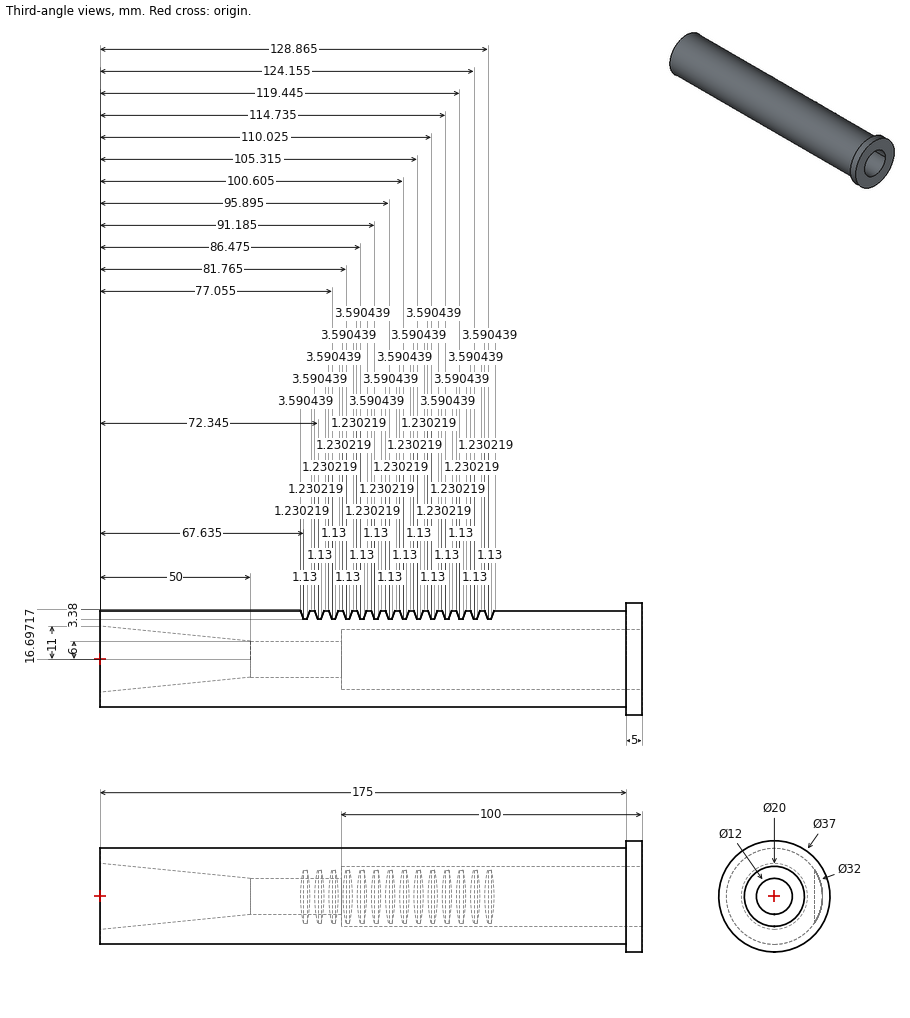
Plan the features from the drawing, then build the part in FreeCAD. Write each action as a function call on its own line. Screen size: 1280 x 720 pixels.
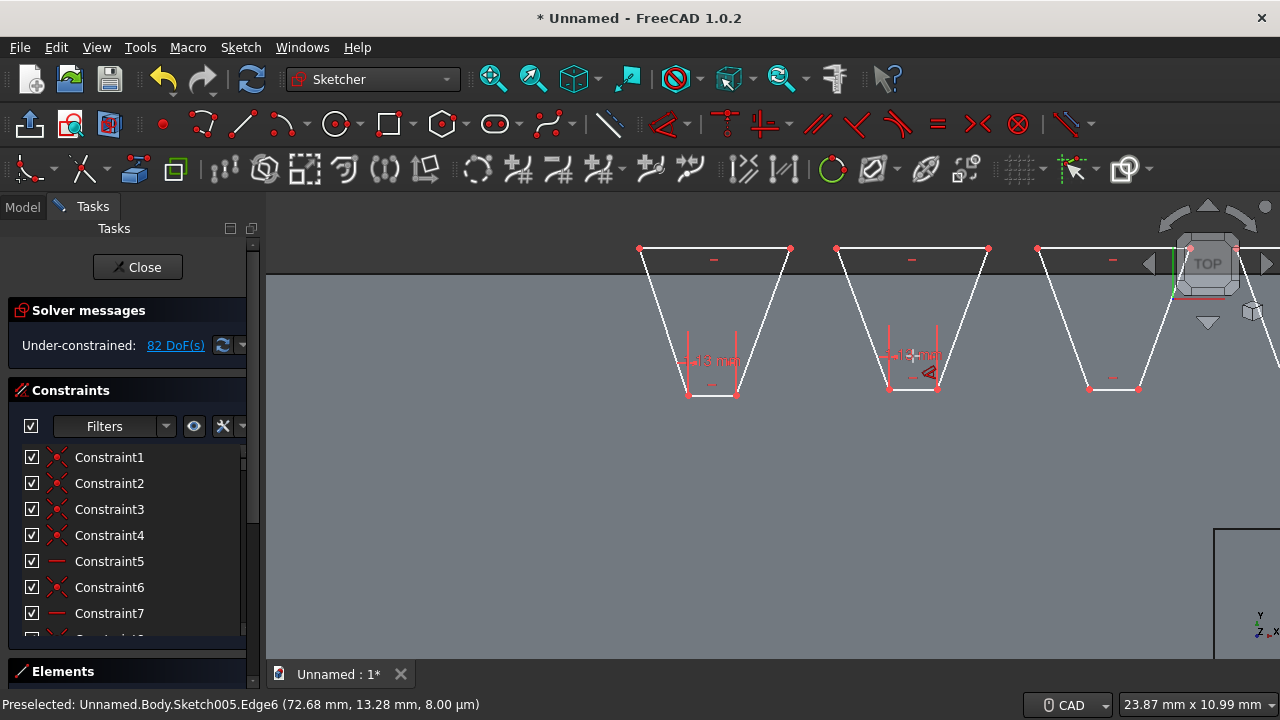
click(1104, 390)
click(1102, 356)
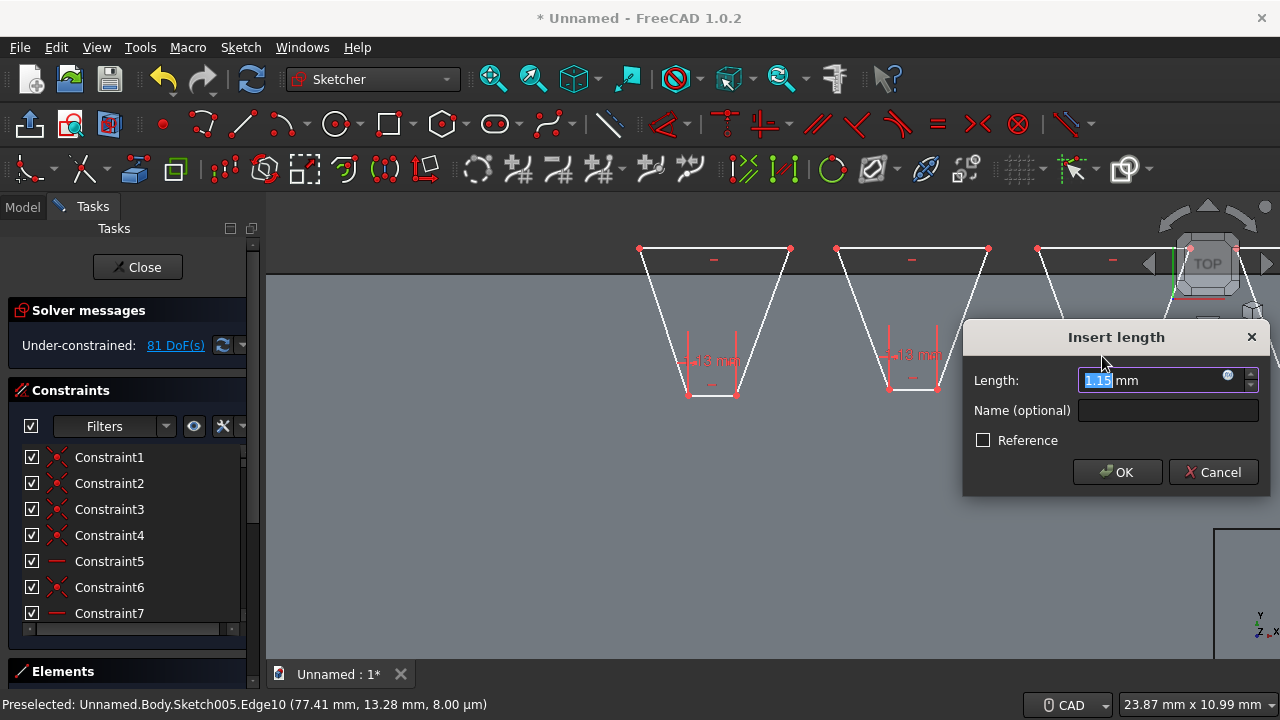
text(1.13)
key(Return)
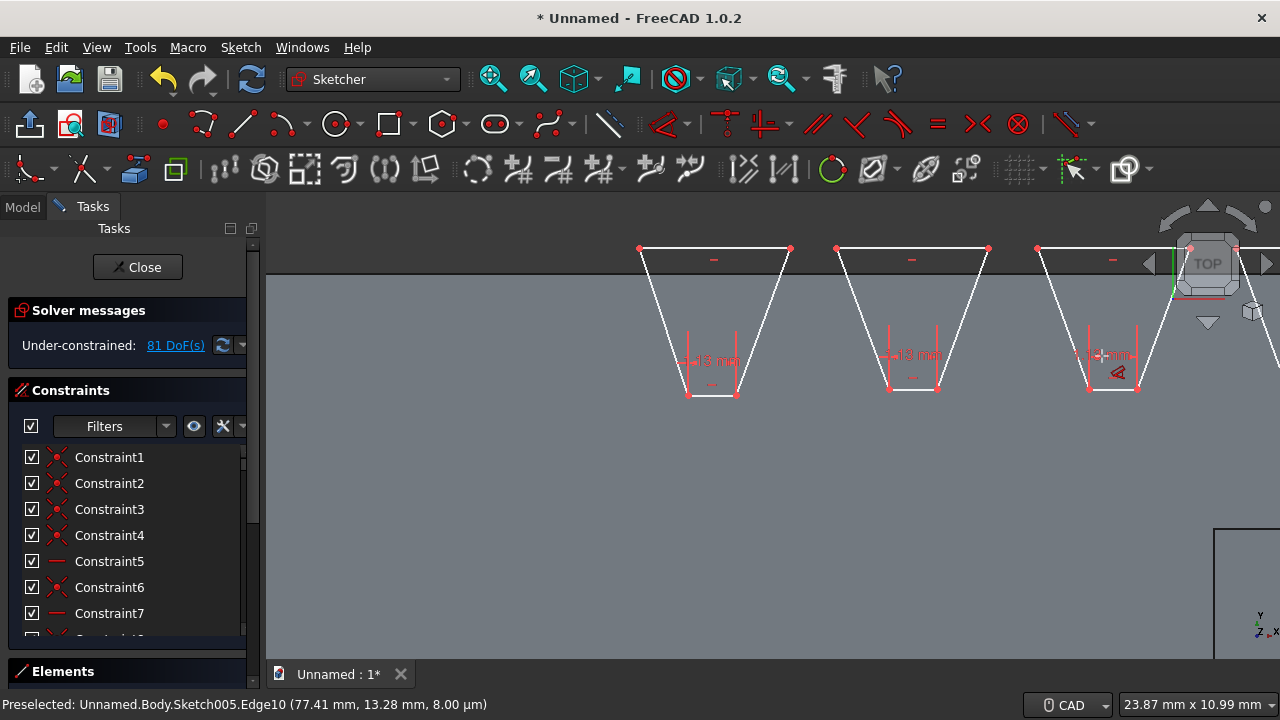
scroll(717, 404, down, 11)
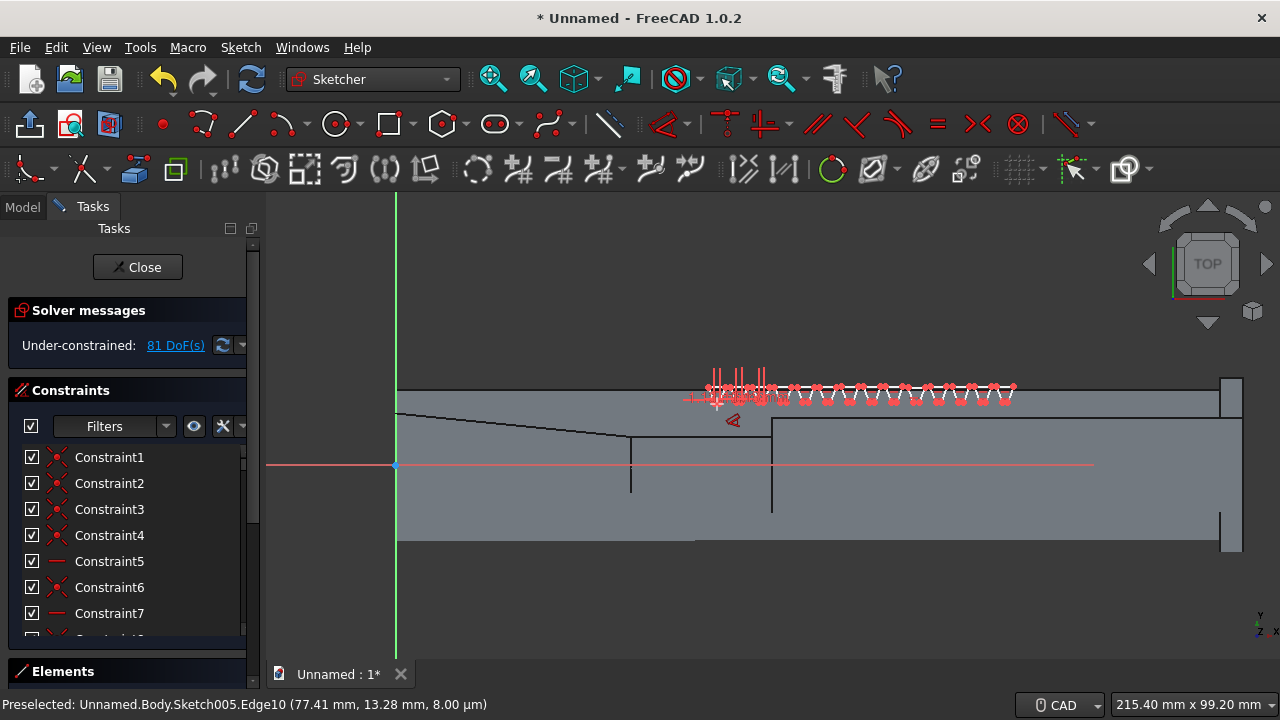
scroll(782, 403, up, 11)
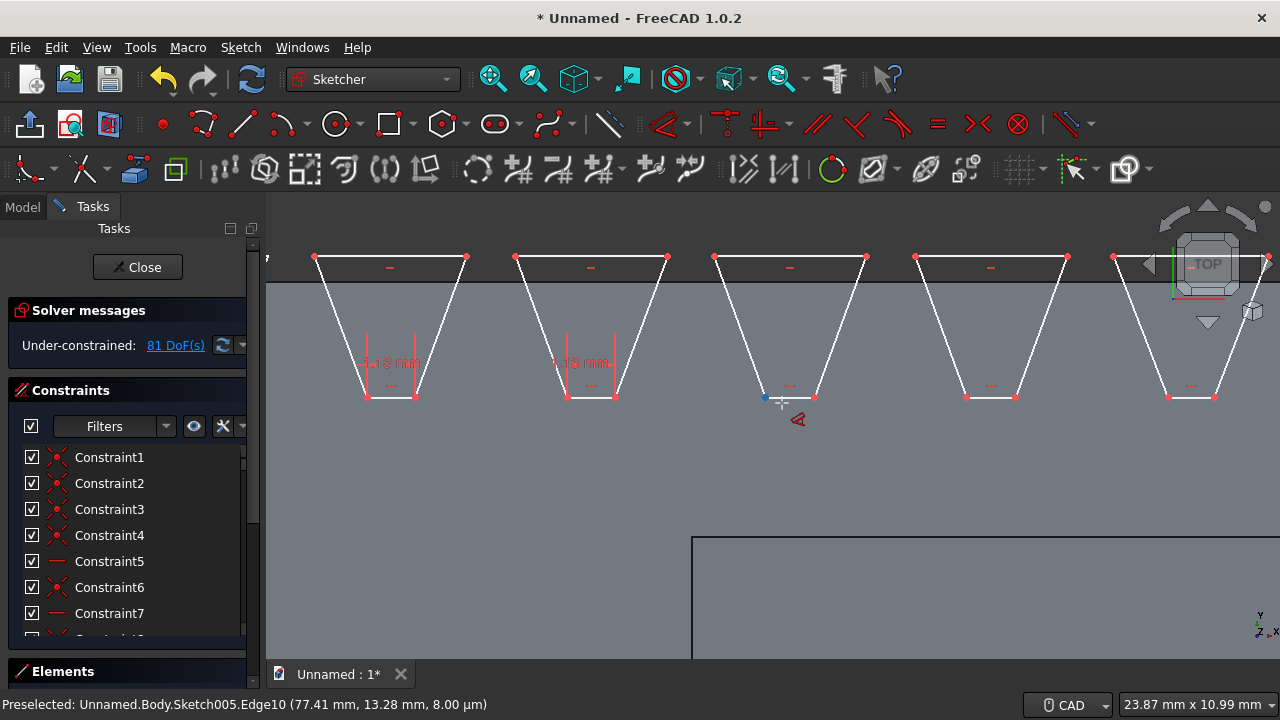
click(780, 398)
click(790, 364)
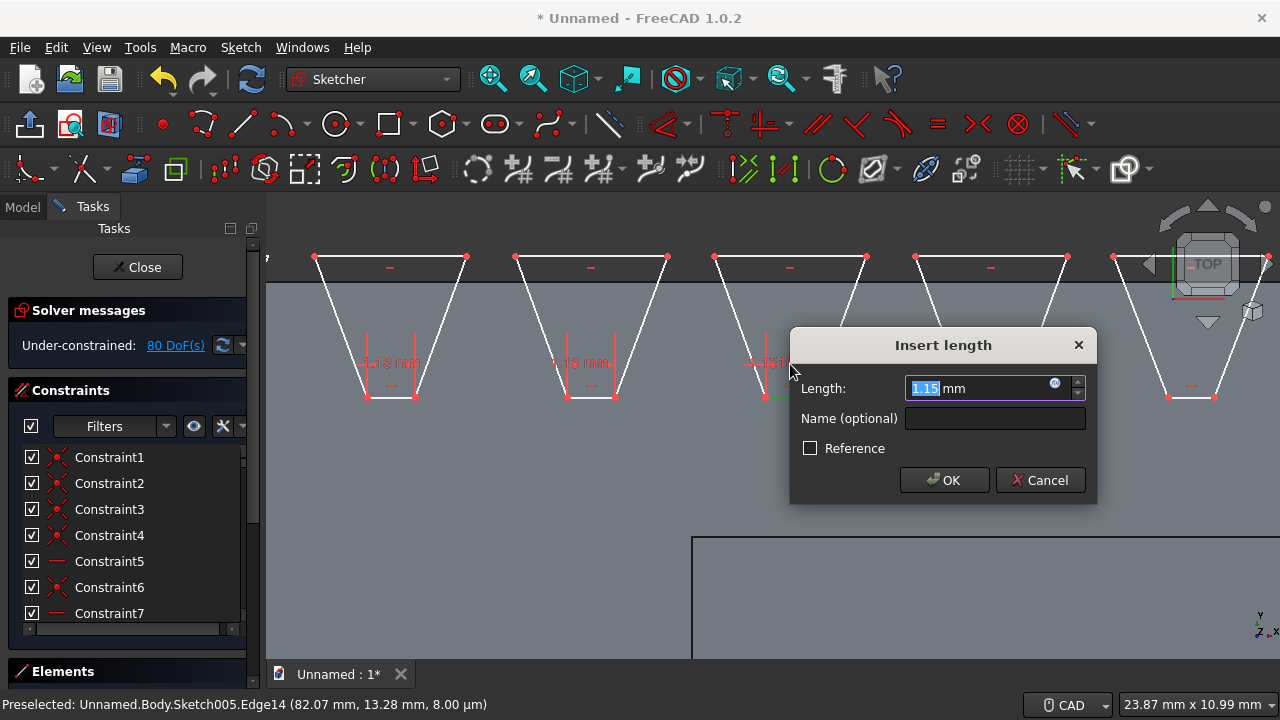
text(1.13)
key(Return)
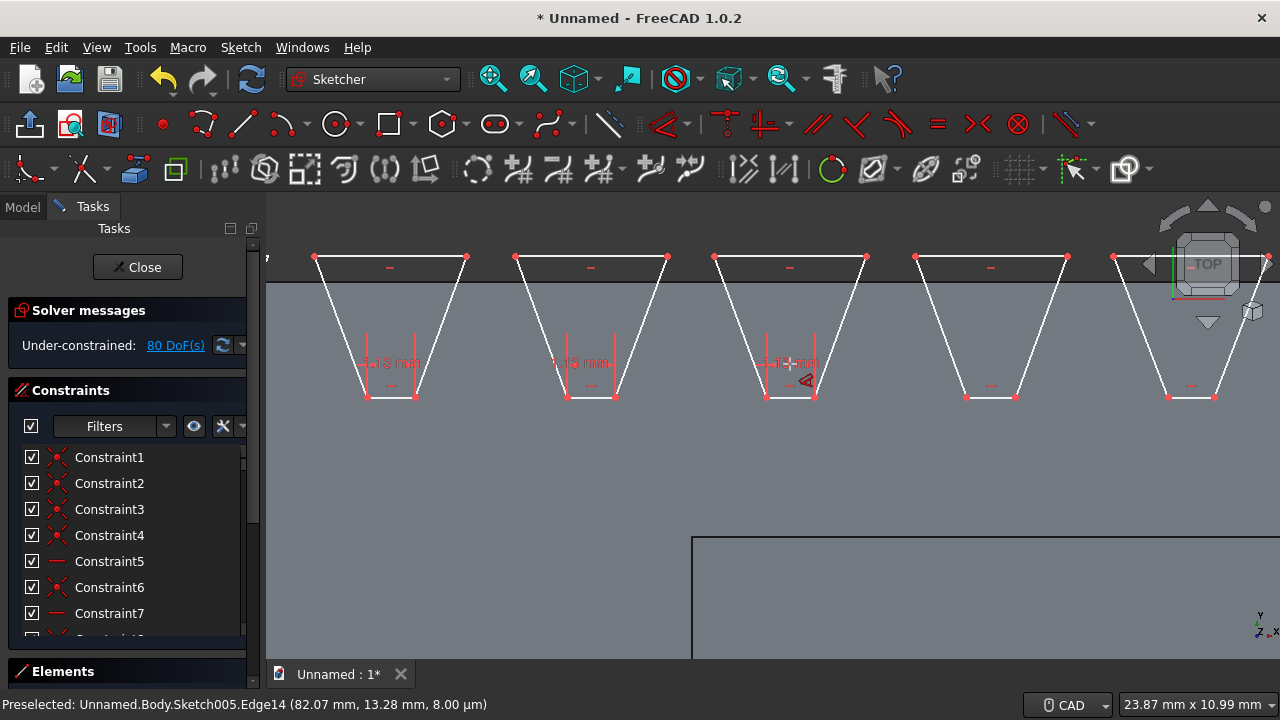
click(982, 398)
click(991, 364)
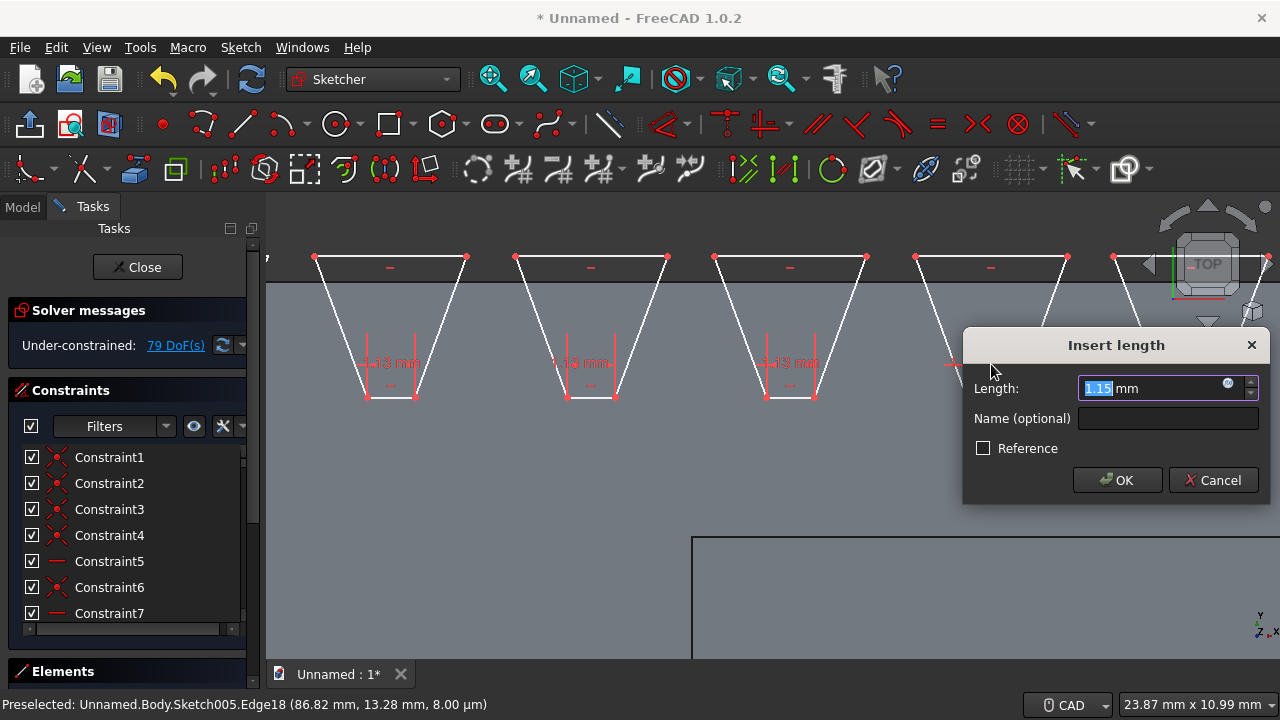
text(1.13)
key(Return)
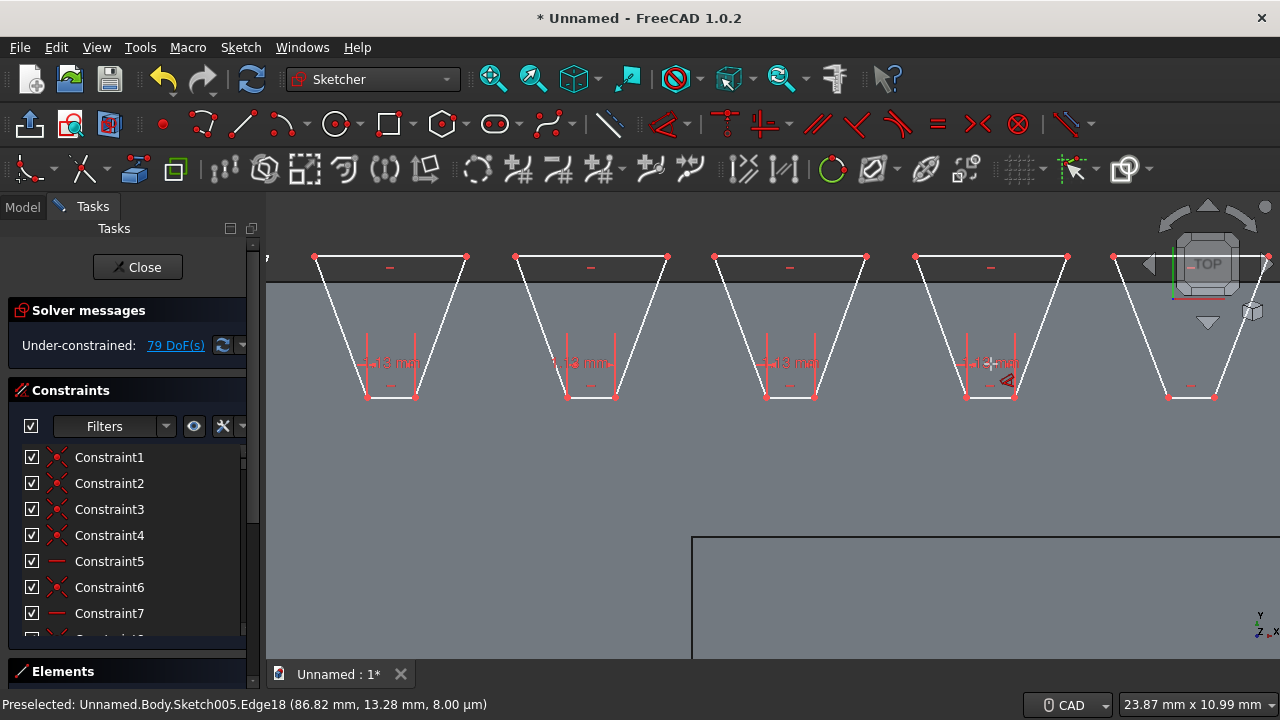
scroll(782, 403, down, 11)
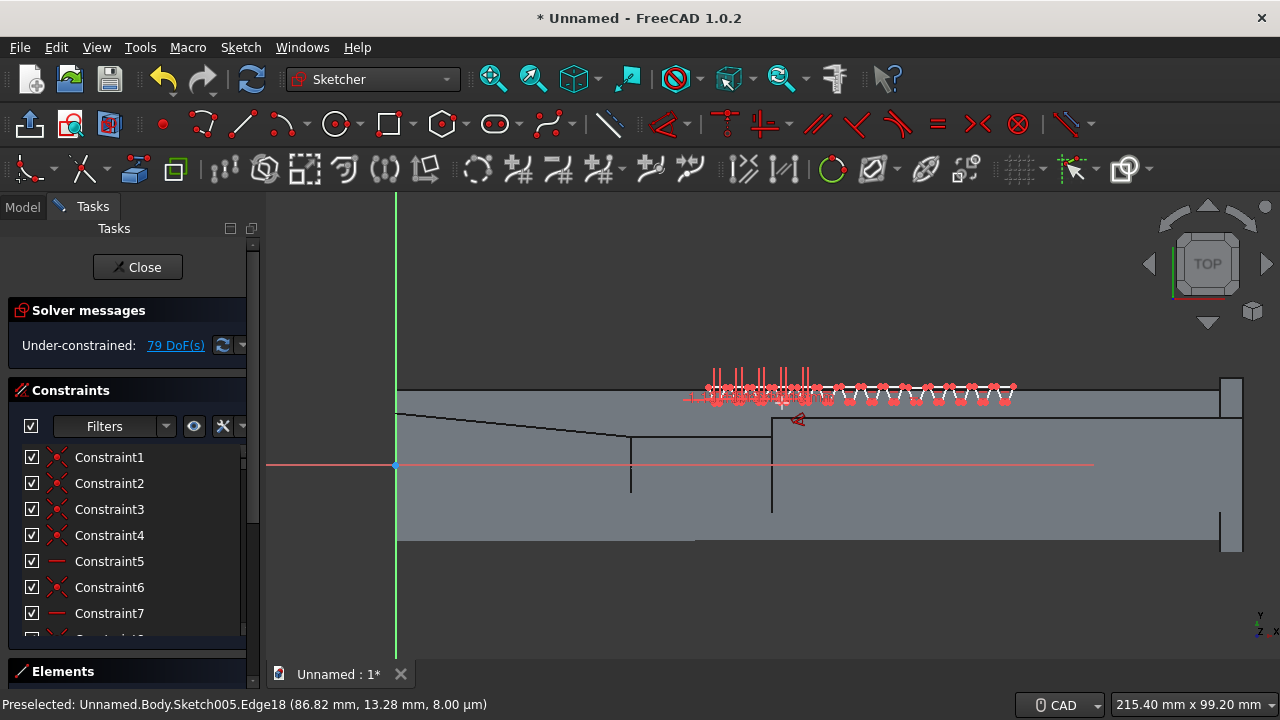
scroll(827, 403, up, 11)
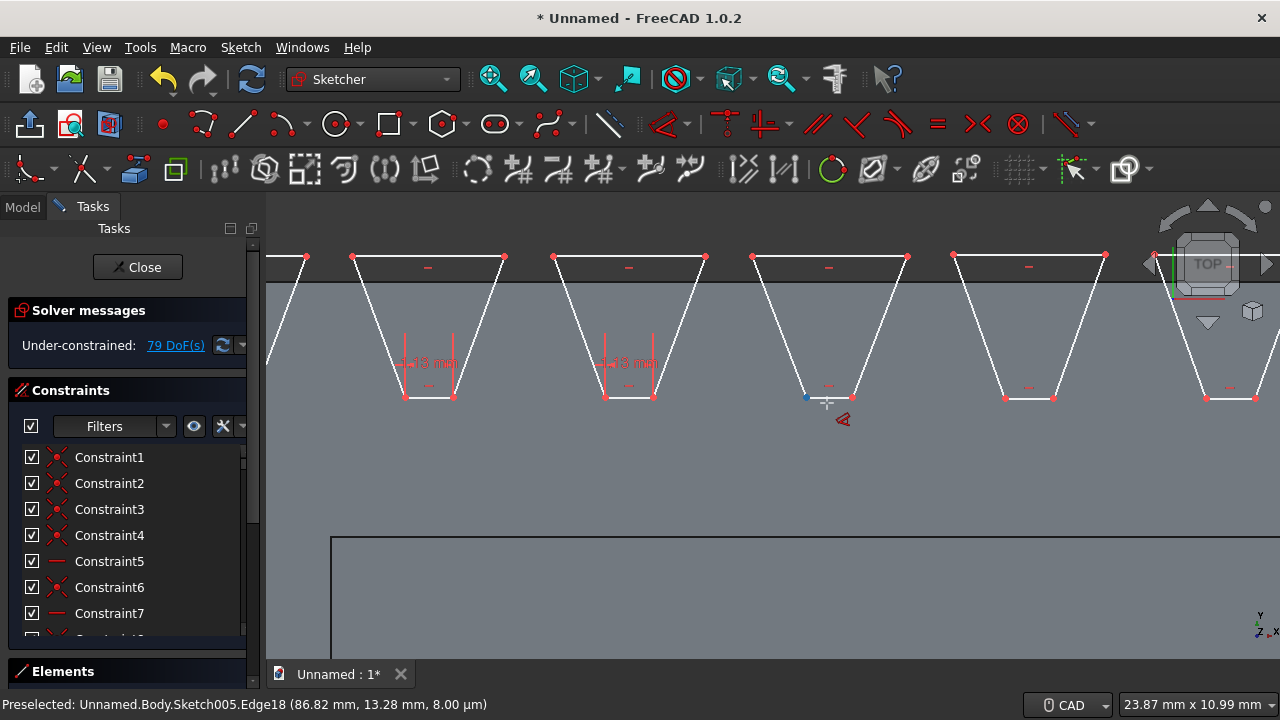
click(820, 398)
click(830, 364)